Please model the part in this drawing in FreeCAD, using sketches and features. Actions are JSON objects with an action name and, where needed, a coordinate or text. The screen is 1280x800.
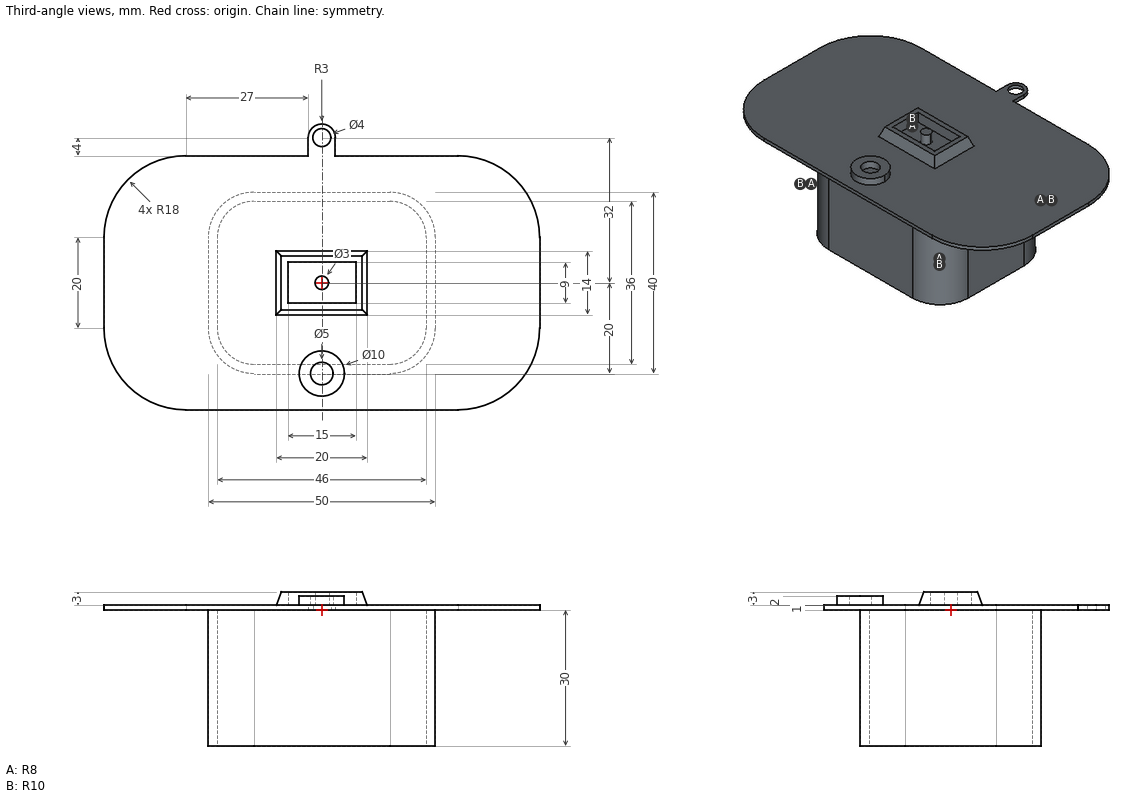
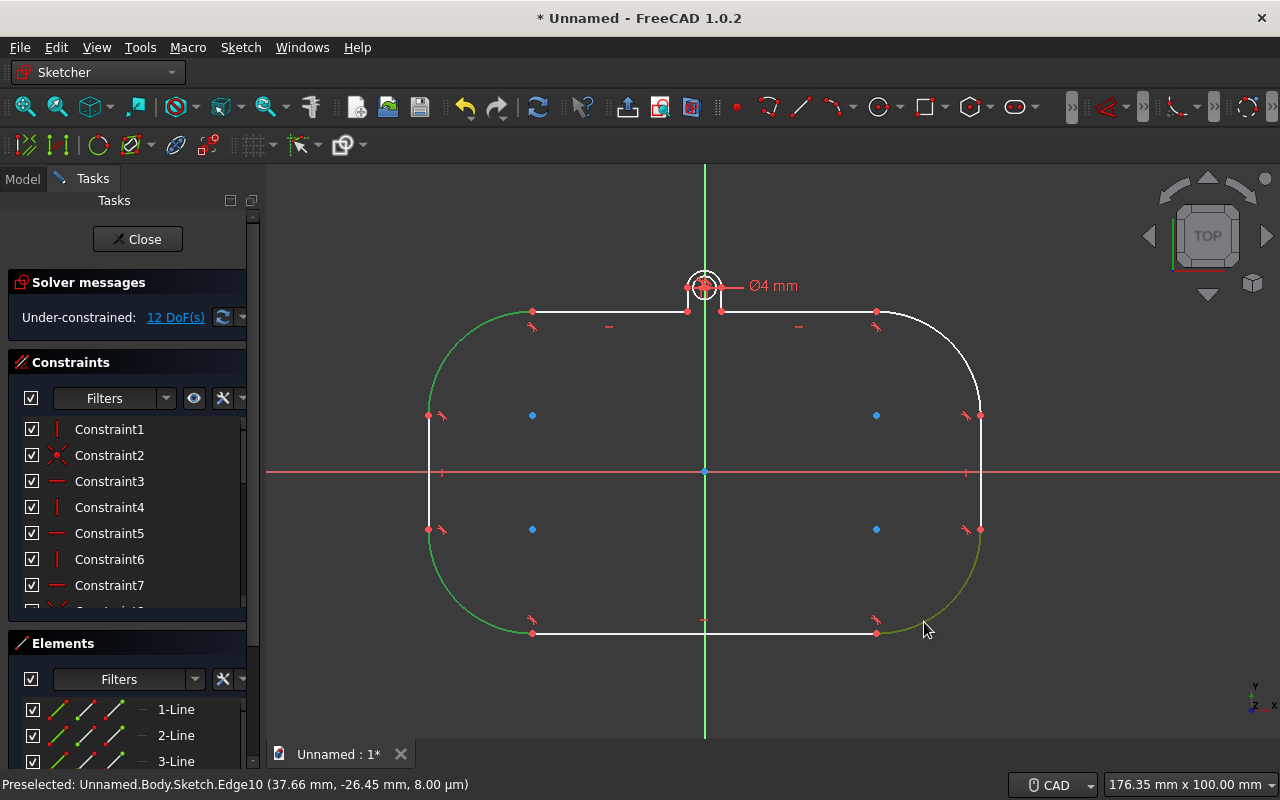
{"action": "left_click", "coordinate": [969, 368]}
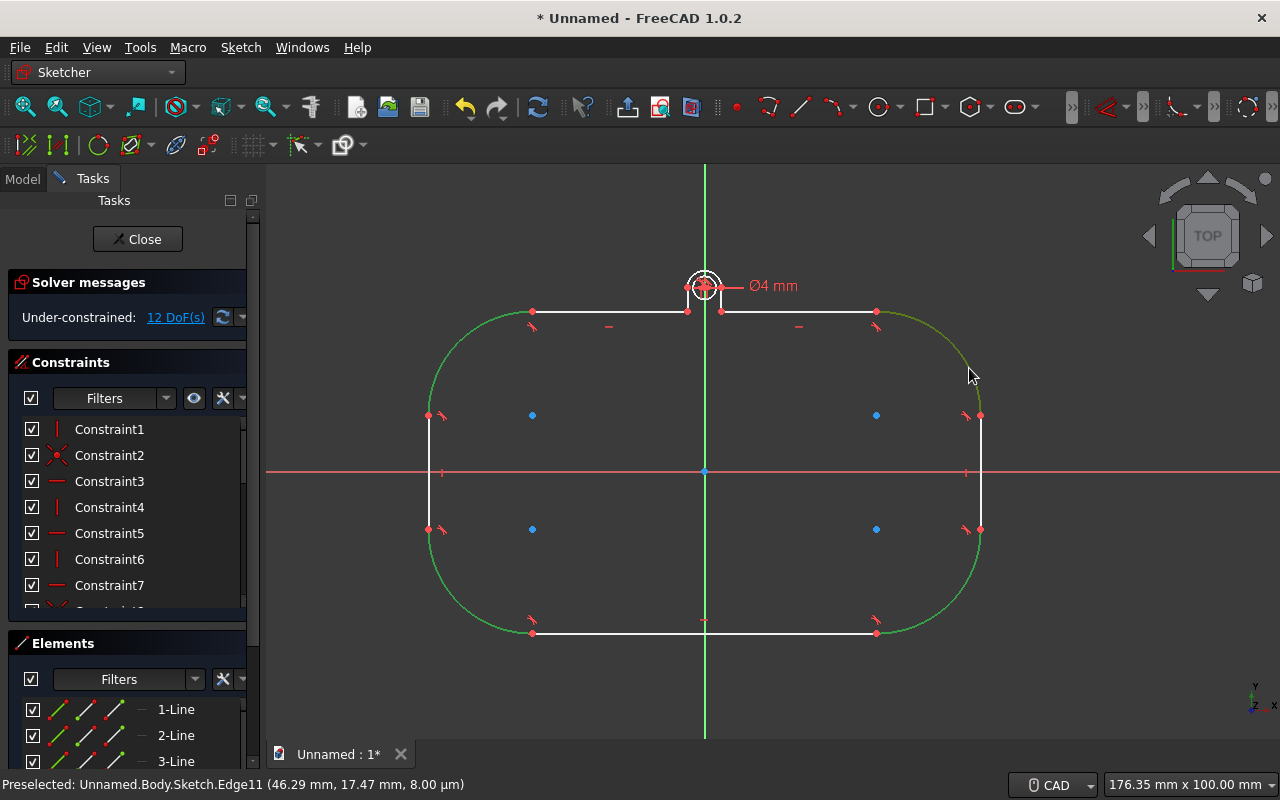
{"action": "key", "text": "e"}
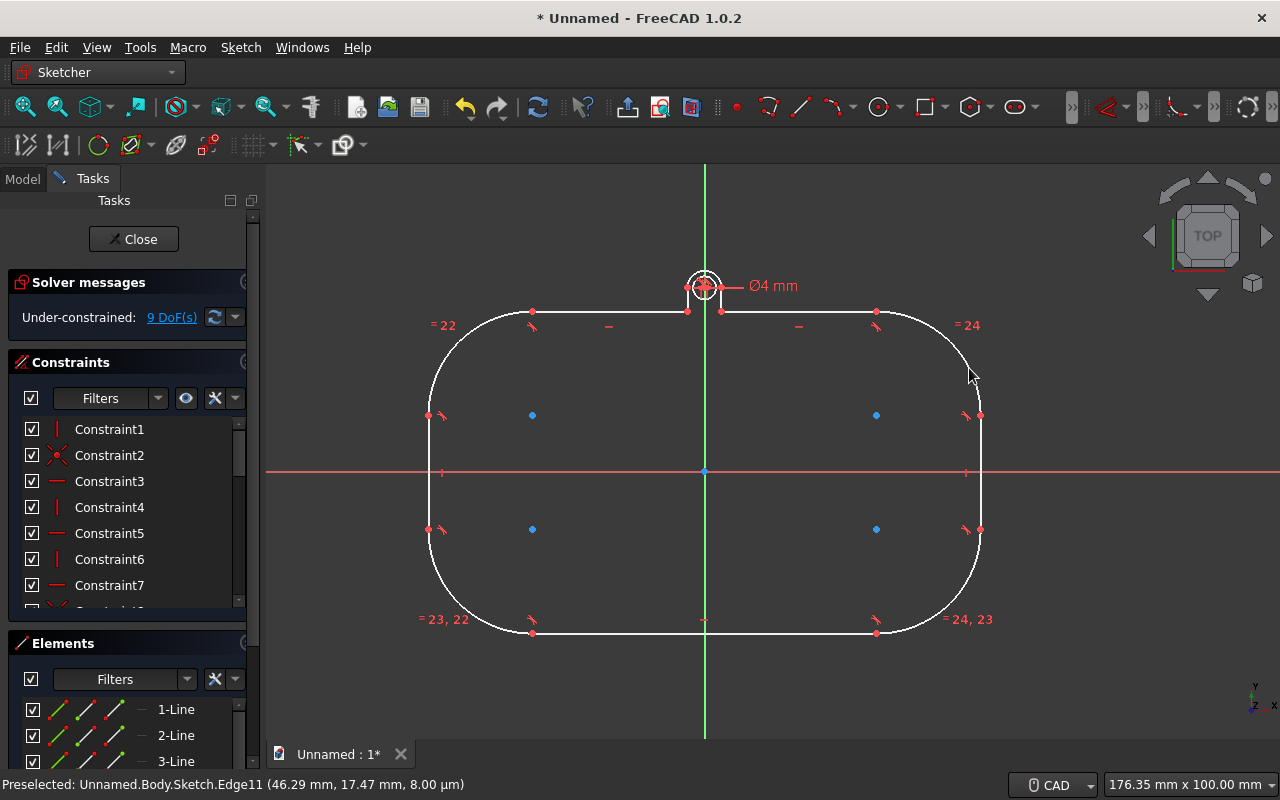
{"action": "left_click", "coordinate": [705, 288]}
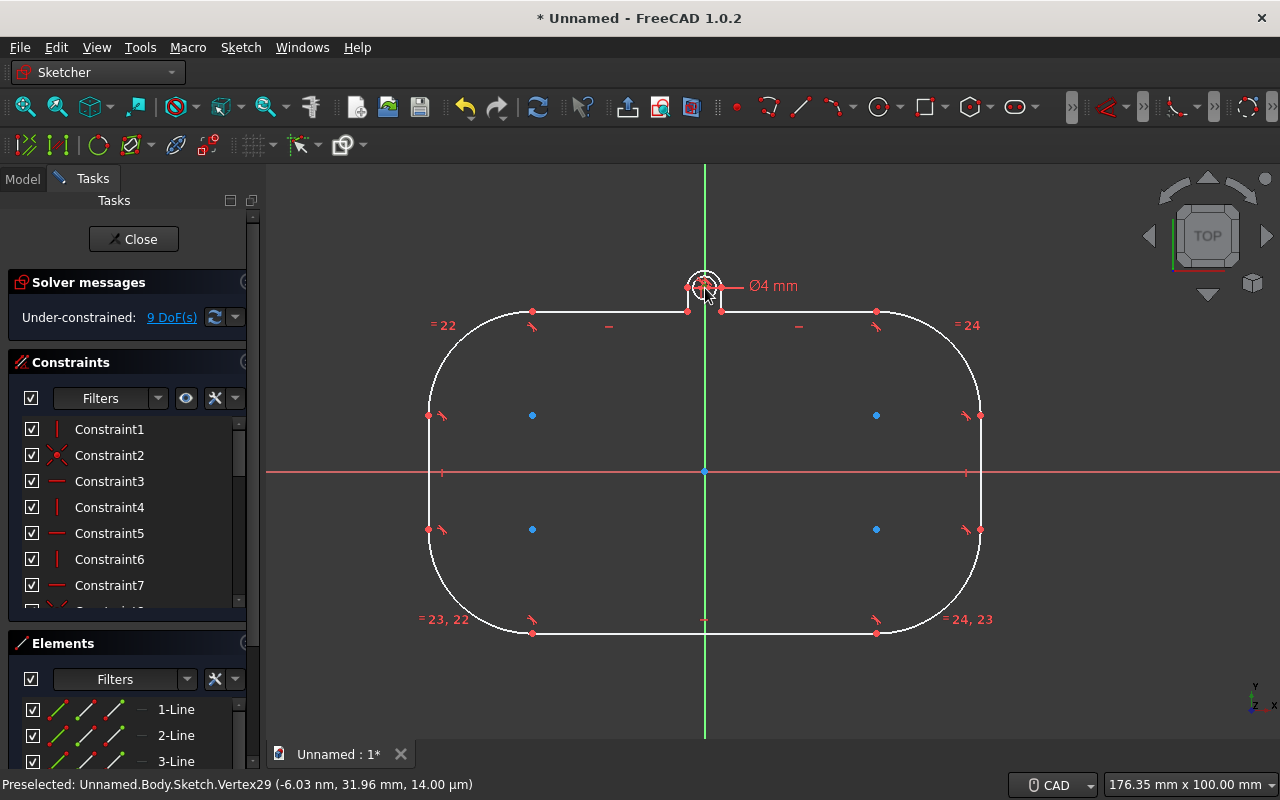
{"action": "left_click", "coordinate": [705, 674]}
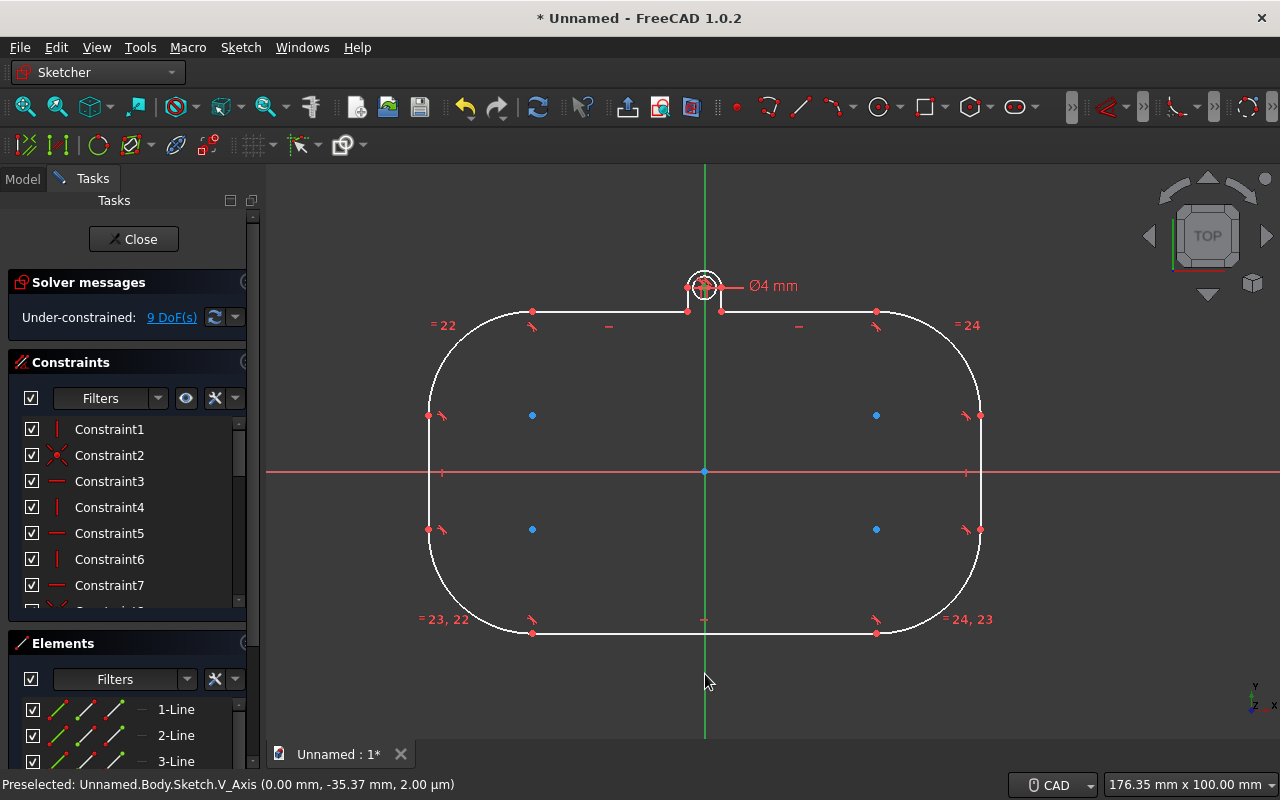
{"action": "key", "text": "c"}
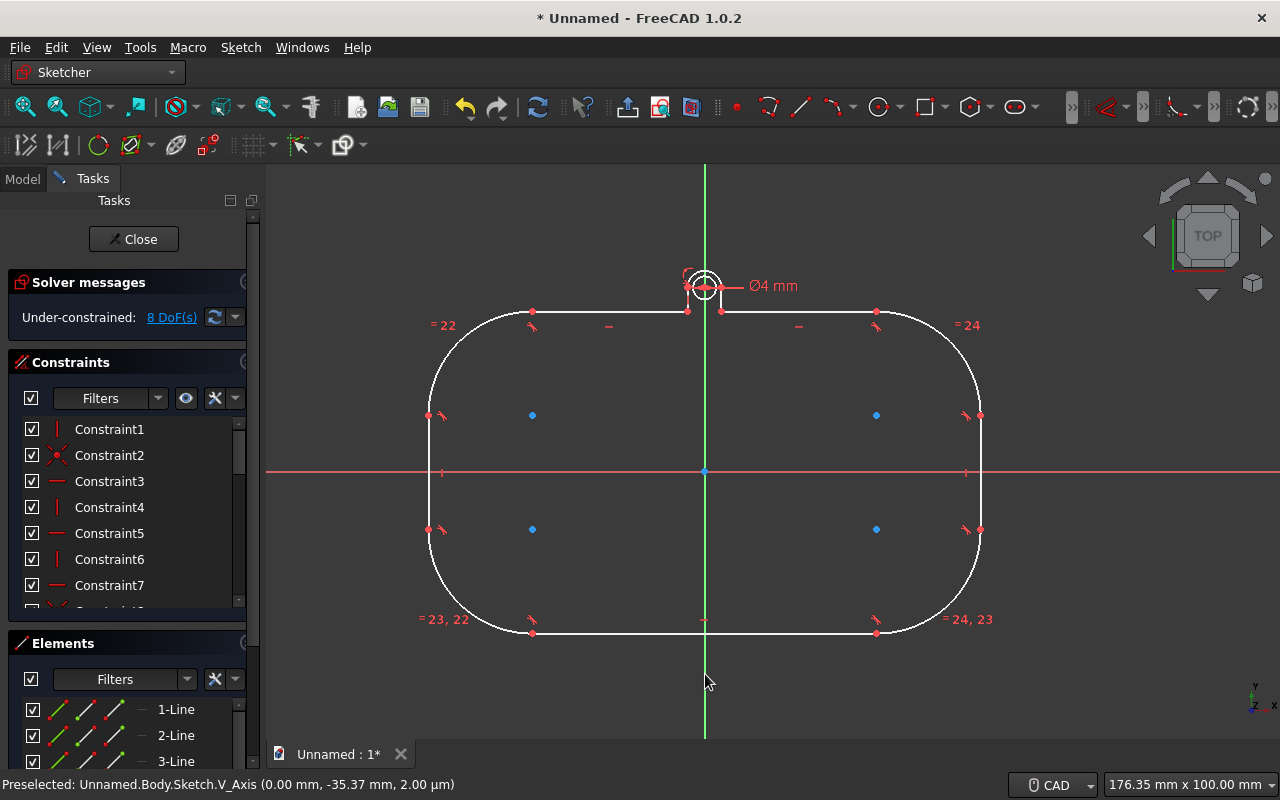
{"action": "left_click", "coordinate": [532, 415]}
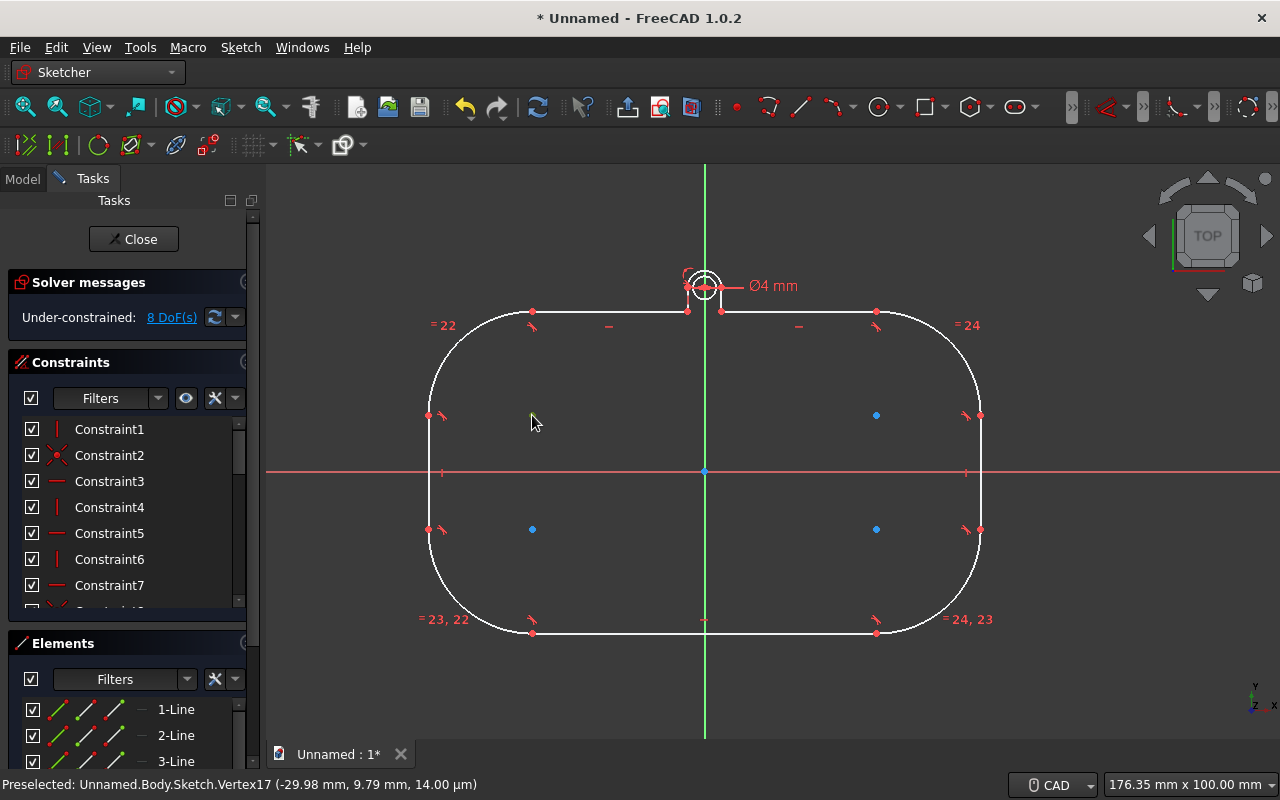
{"action": "left_click", "coordinate": [877, 415]}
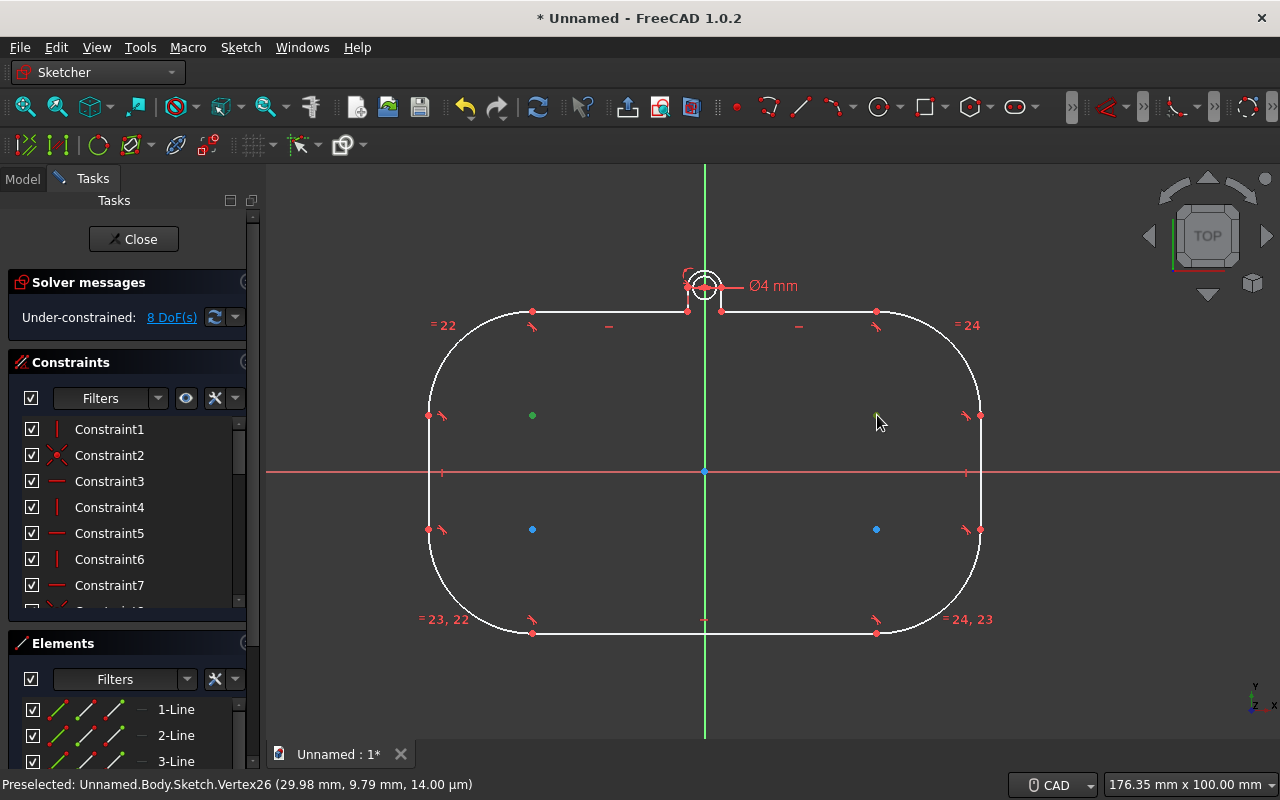
{"action": "left_click", "coordinate": [705, 674]}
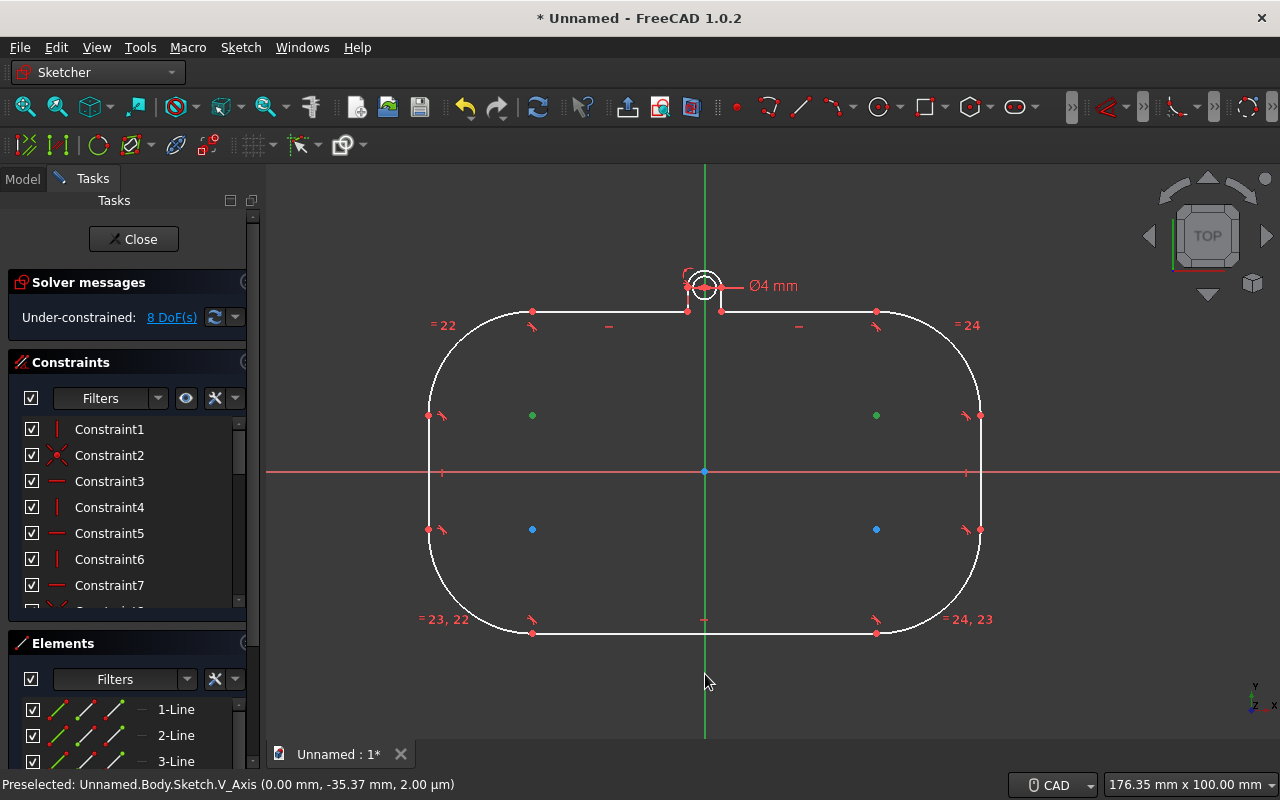
{"action": "key", "text": "s"}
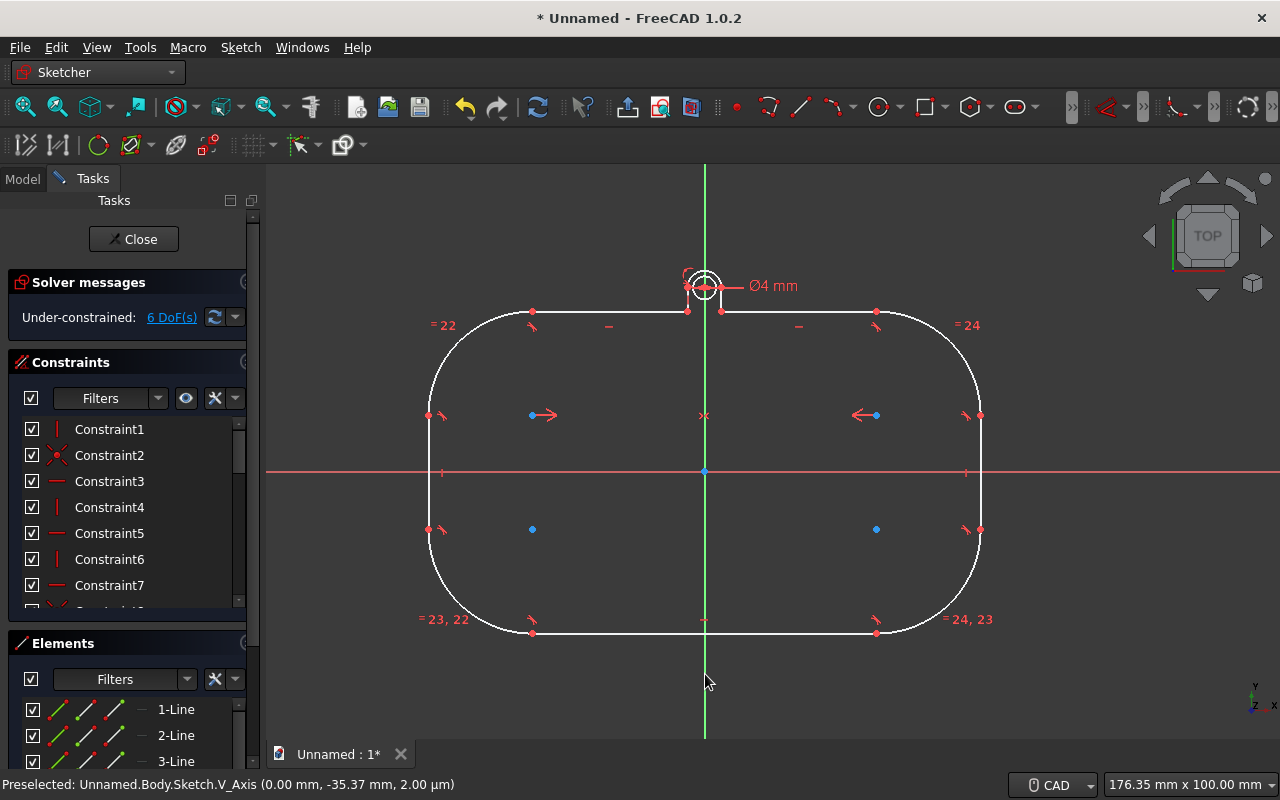
{"action": "left_click", "coordinate": [1106, 108]}